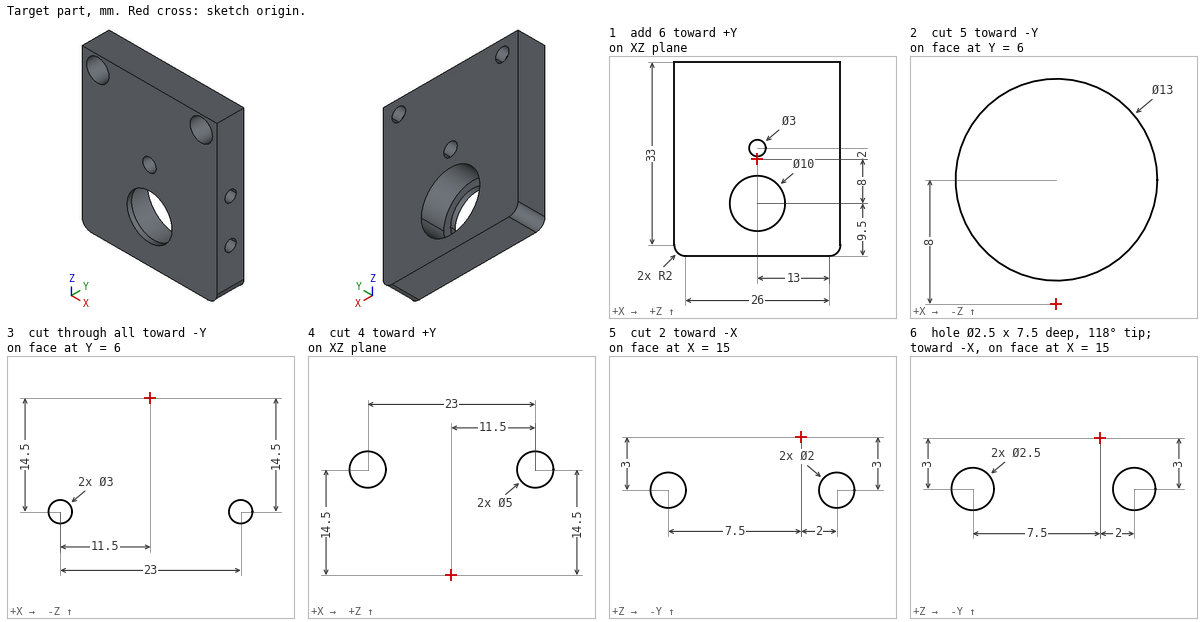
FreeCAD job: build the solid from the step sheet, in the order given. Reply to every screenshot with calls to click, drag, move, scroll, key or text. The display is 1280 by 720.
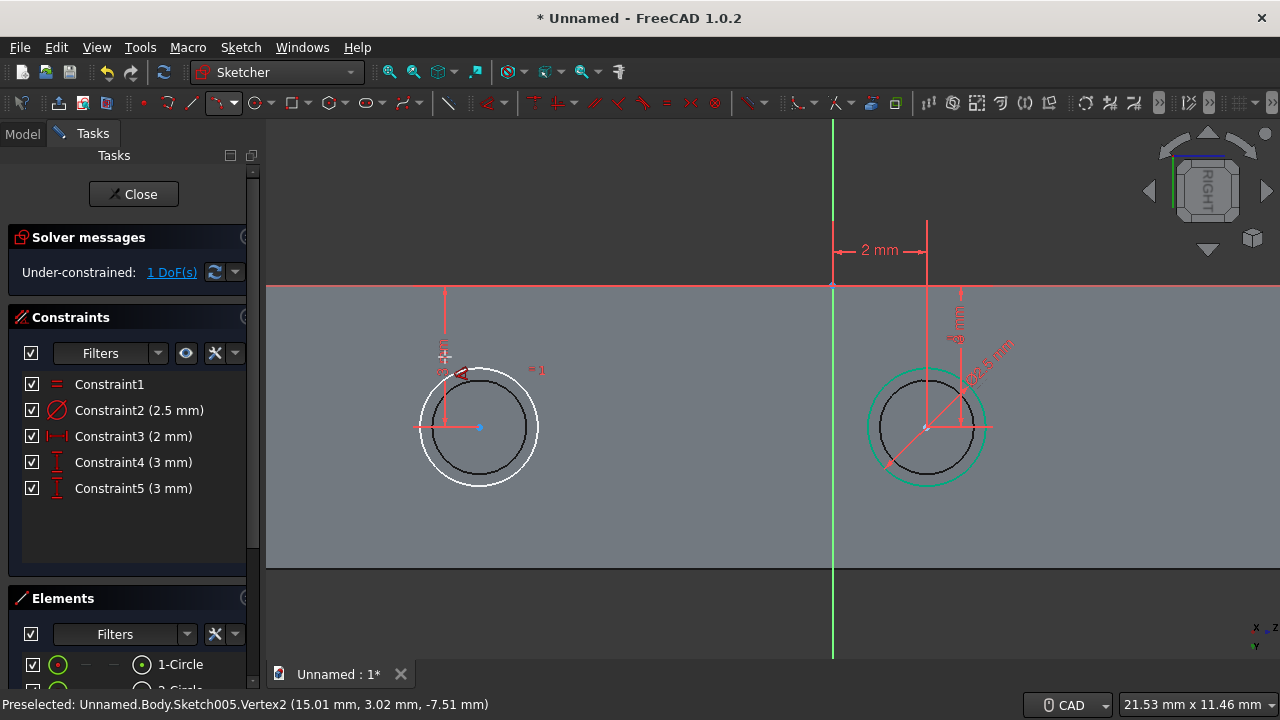
click(479, 427)
click(656, 252)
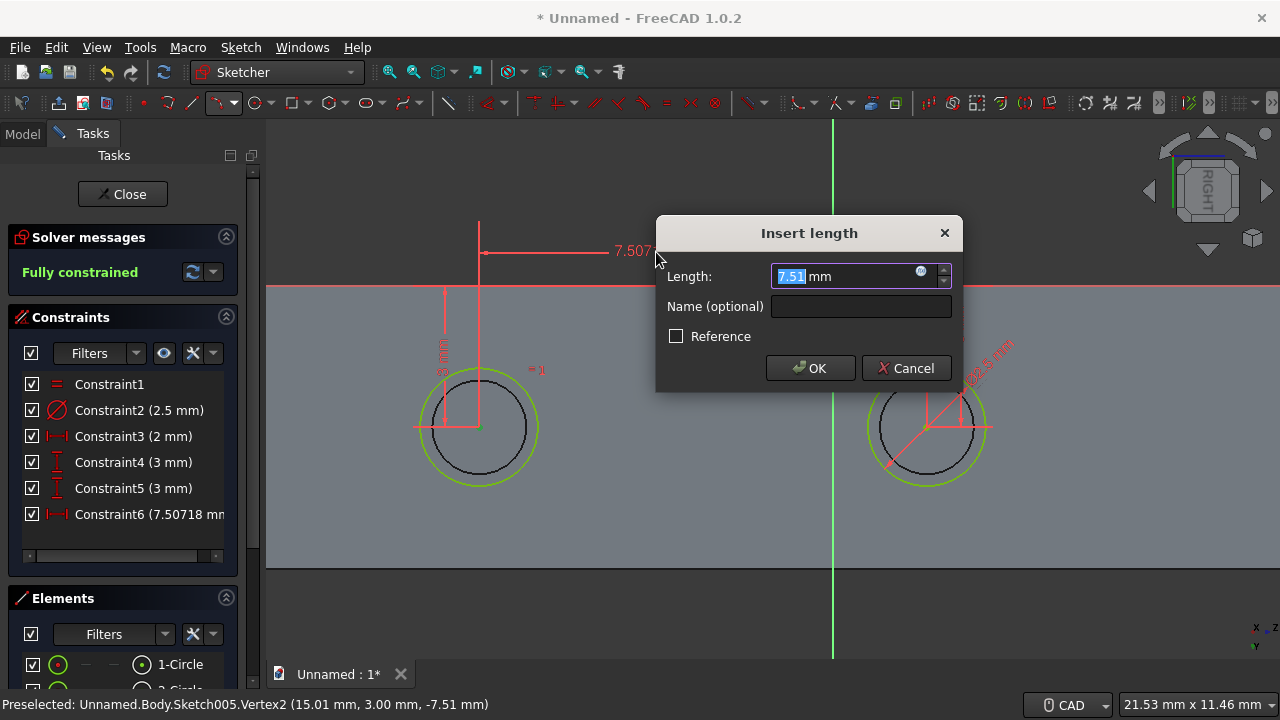
text(7.5)
key(Return)
key(Escape)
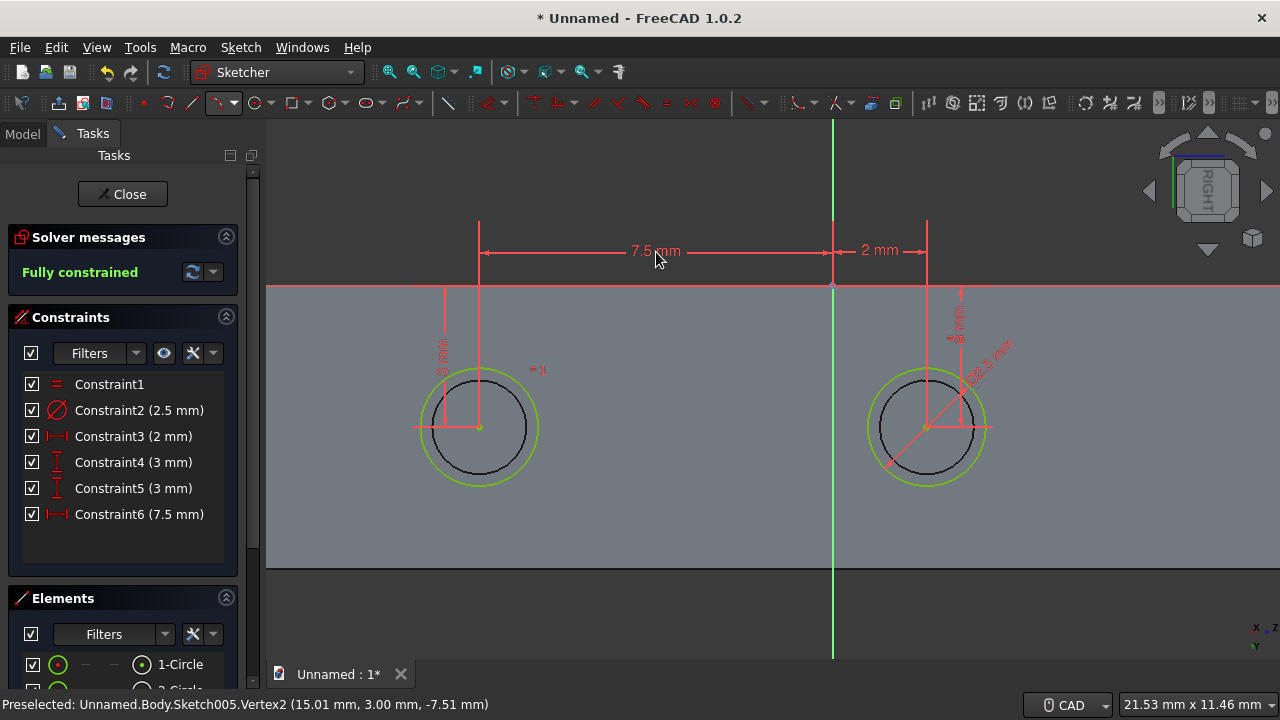
click(123, 194)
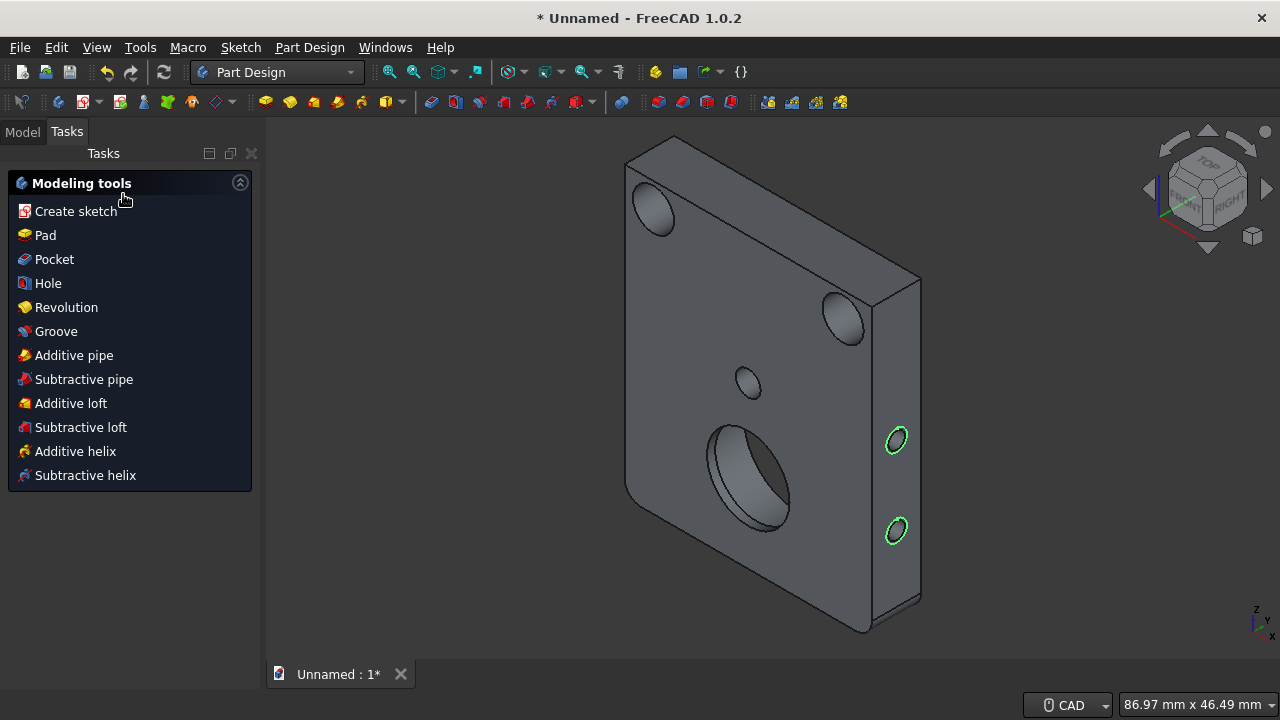
click(456, 102)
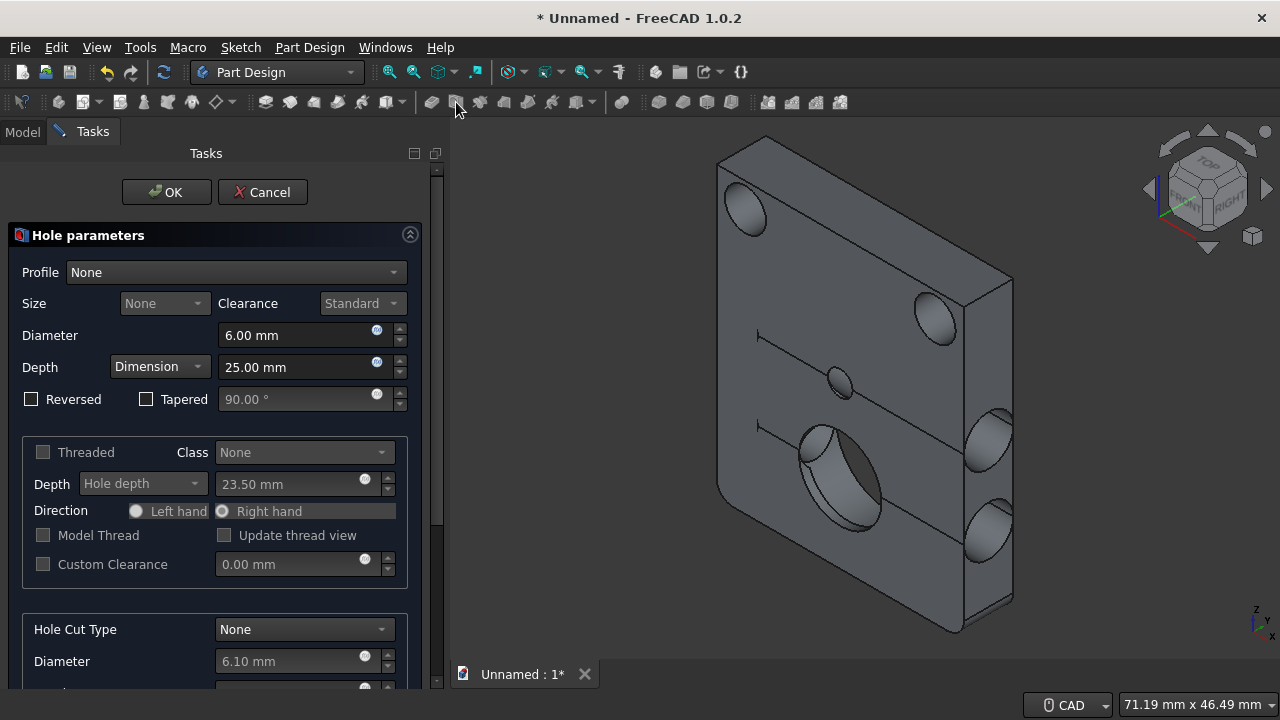
triple_click(305, 335)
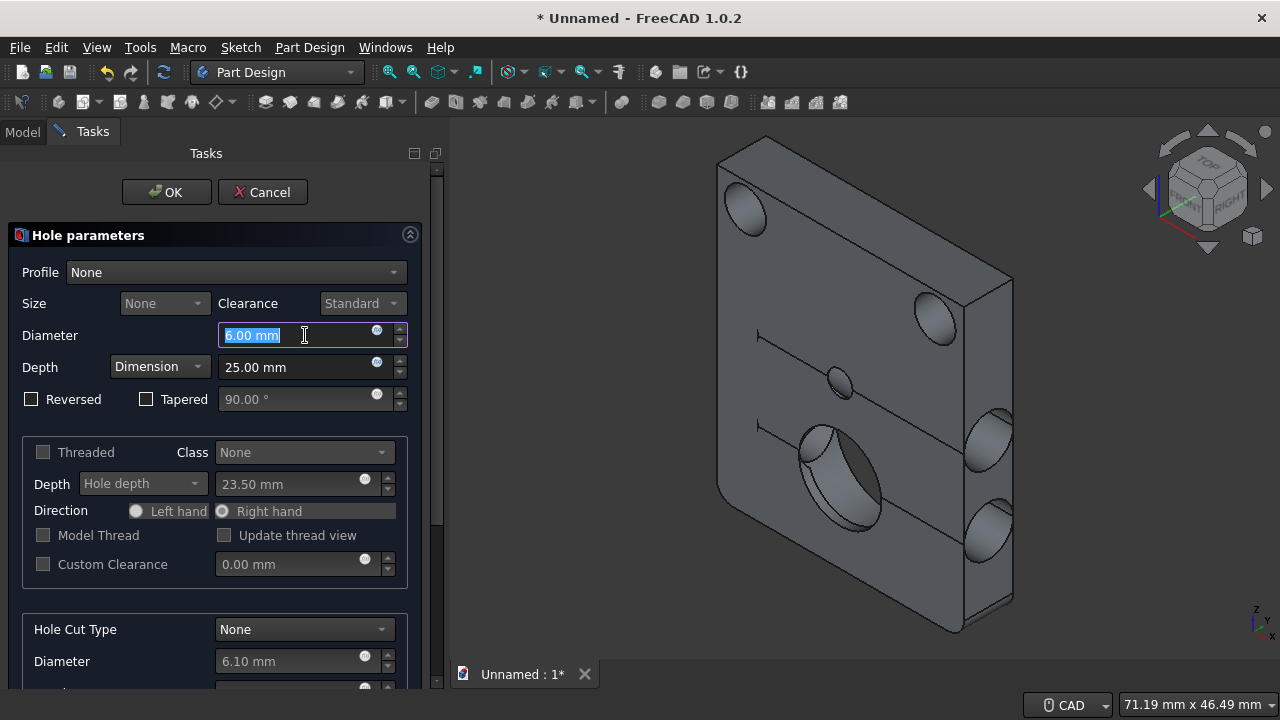
text(2.5)
key(Tab)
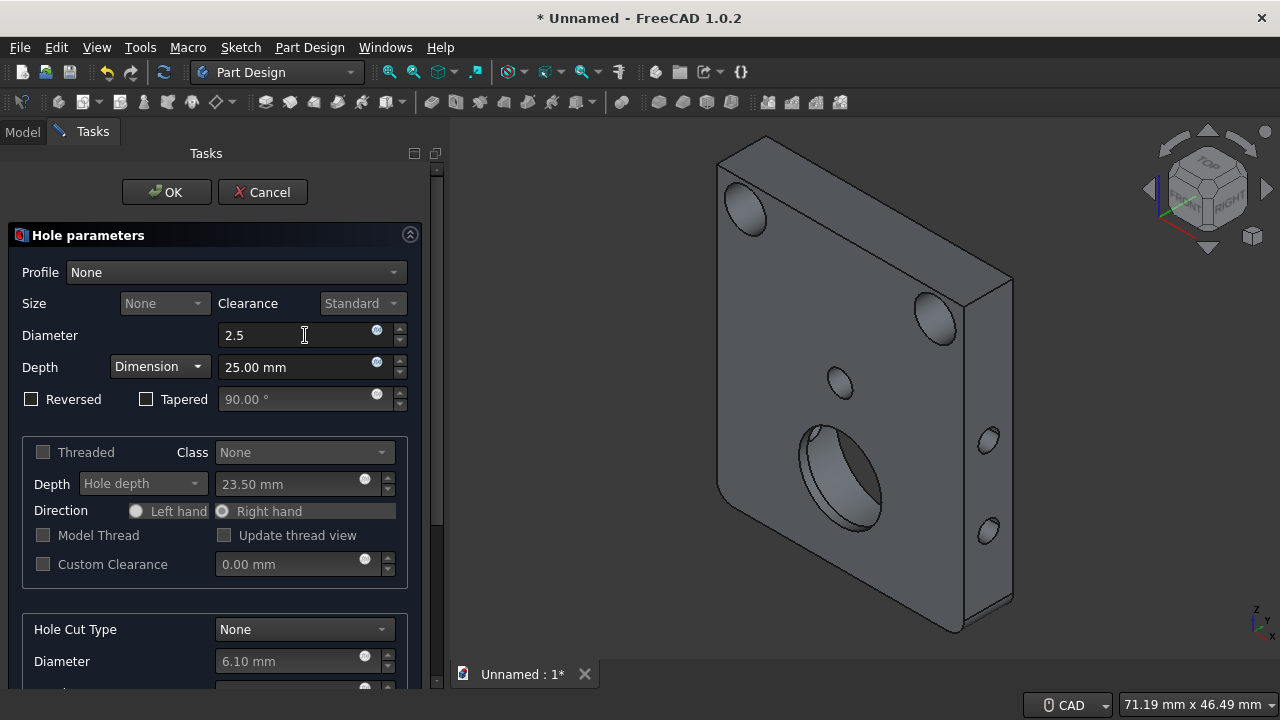
triple_click(305, 367)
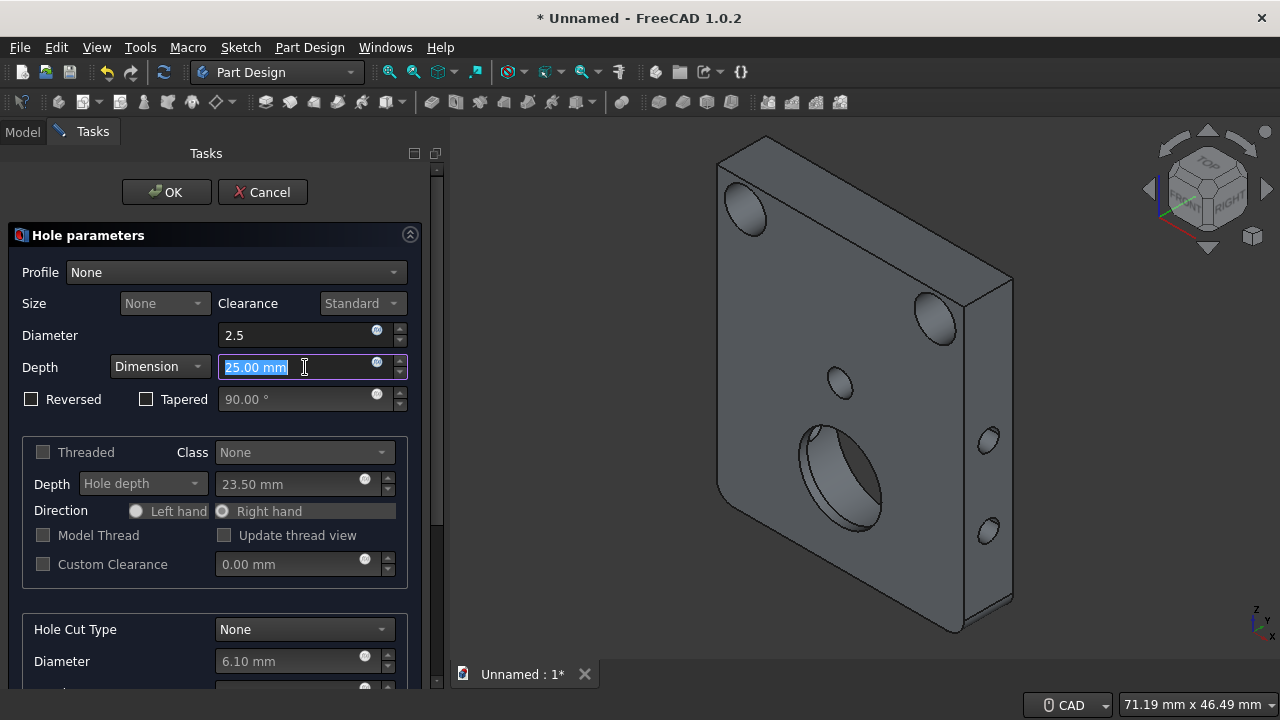
text(7.5)
key(Tab)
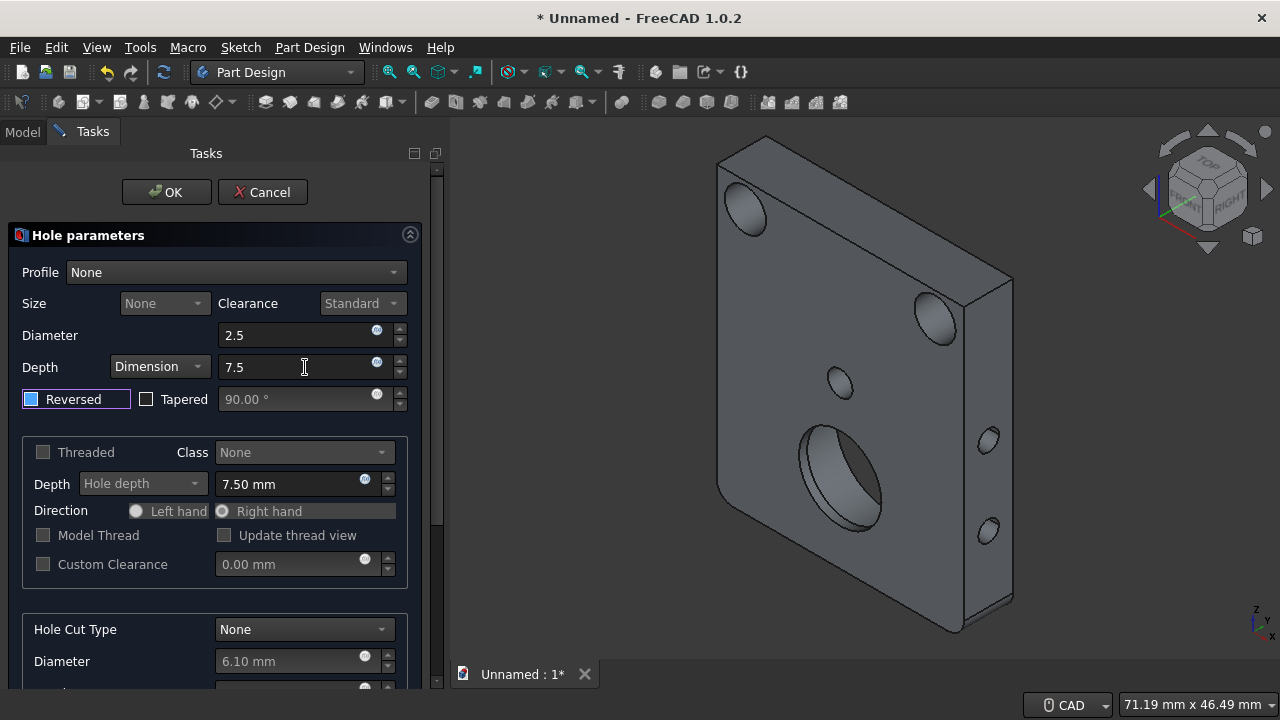
click(167, 192)